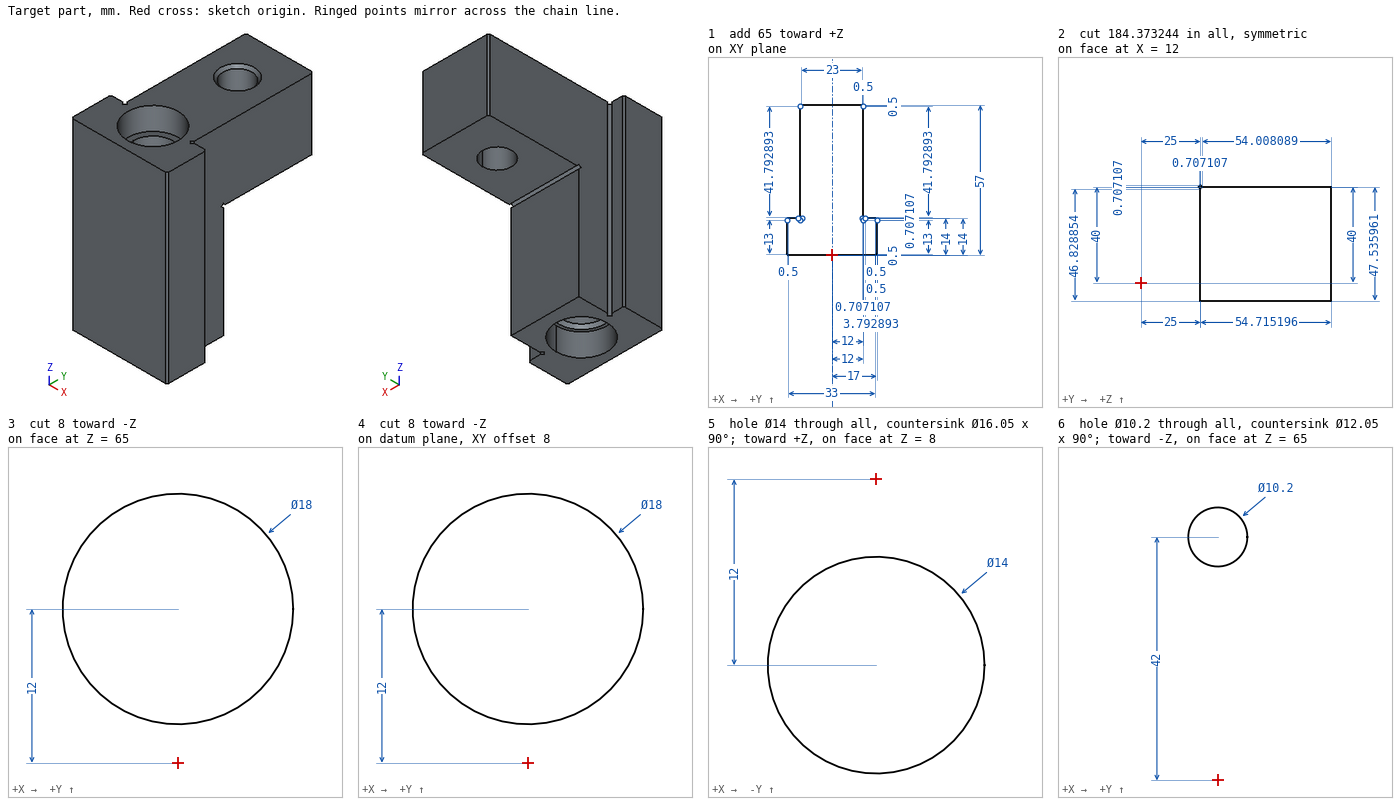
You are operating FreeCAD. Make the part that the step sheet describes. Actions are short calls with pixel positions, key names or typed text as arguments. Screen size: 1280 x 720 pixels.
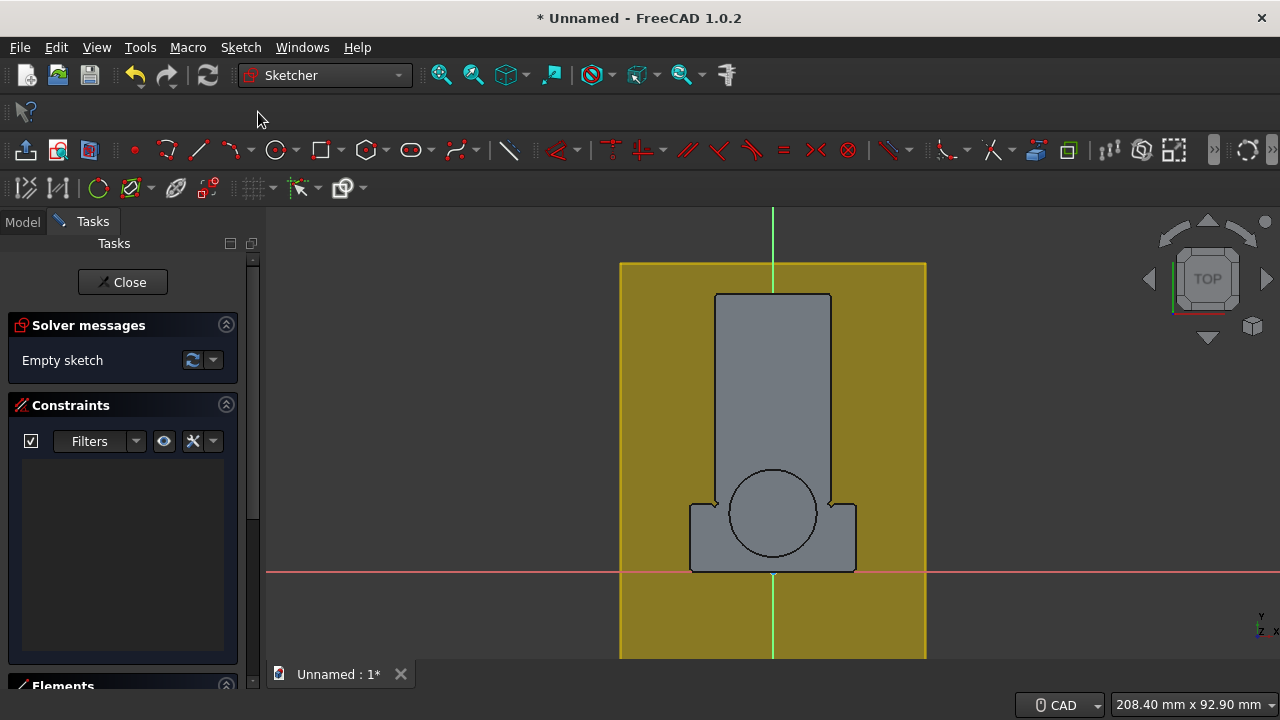
click(90, 150)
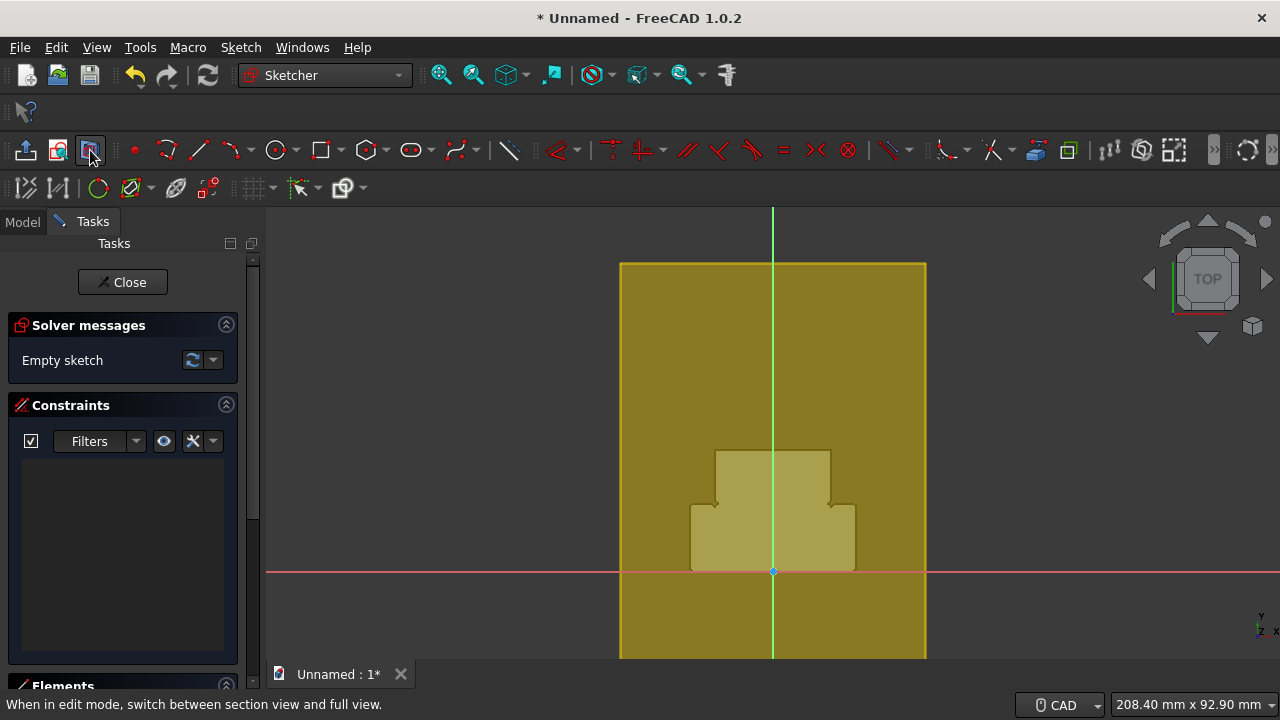
scroll(813, 572, up, 5)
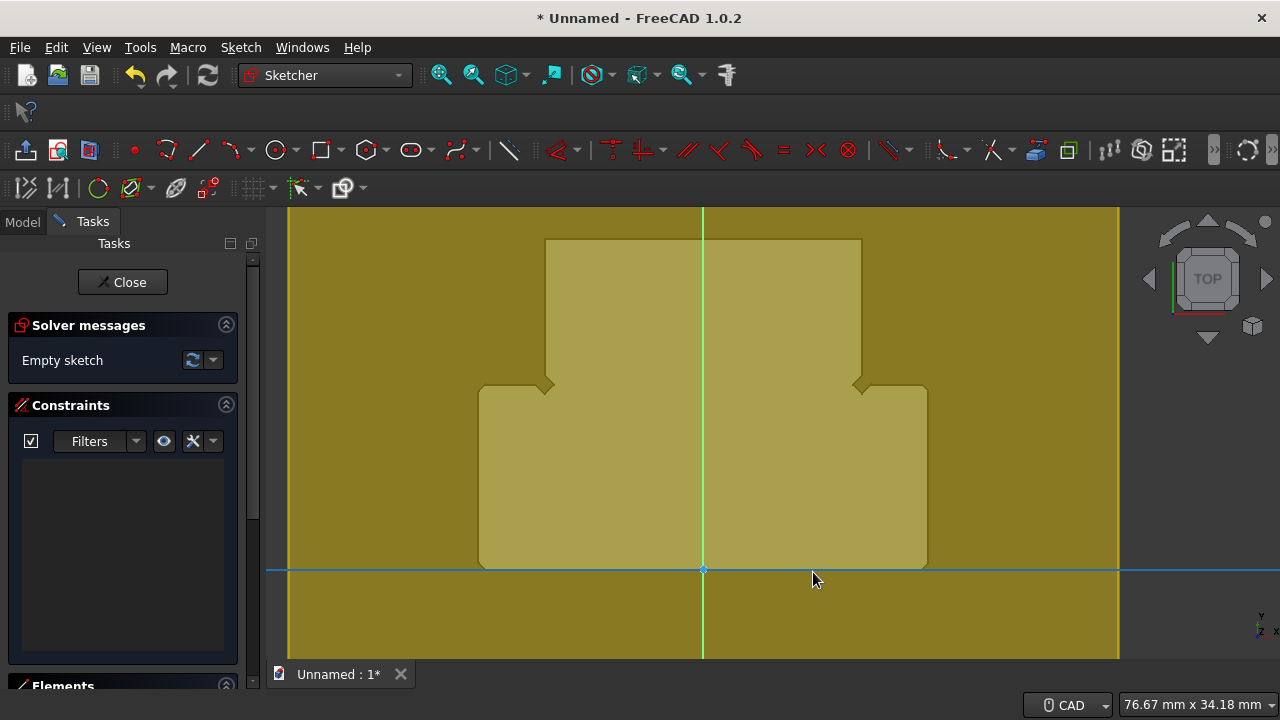
key(g)
key(c)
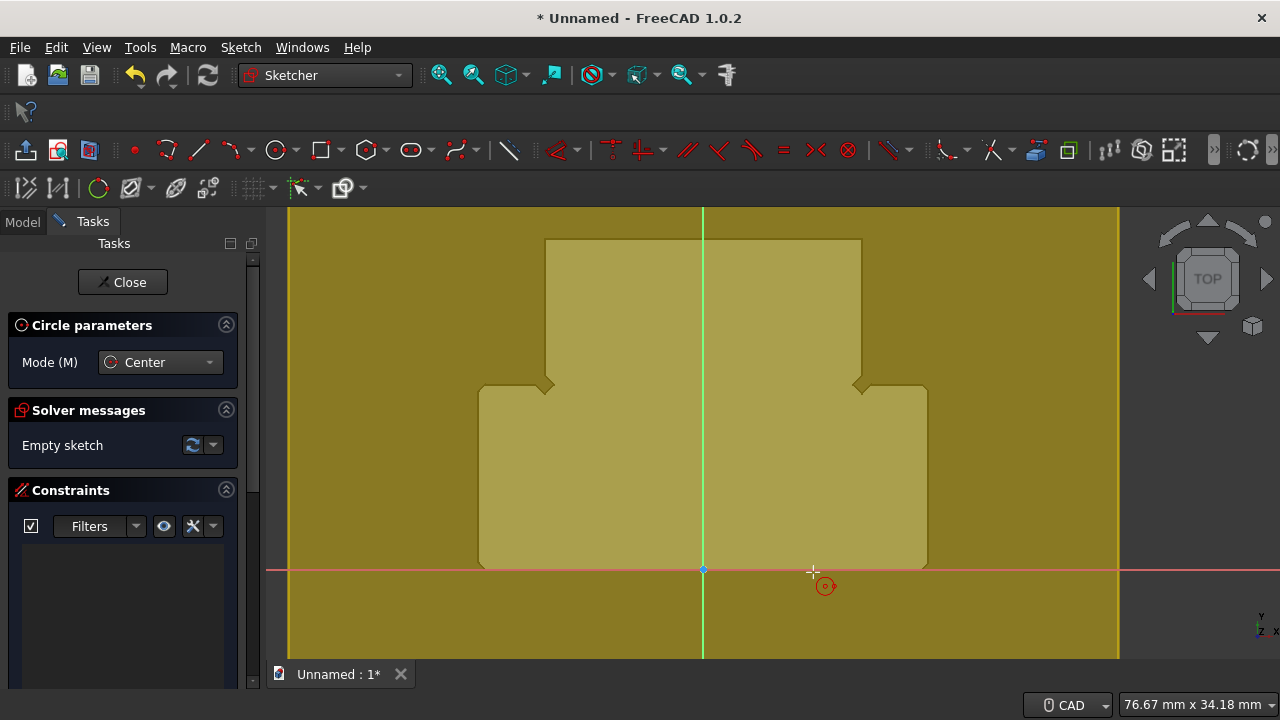
click(703, 411)
click(788, 327)
key(Escape)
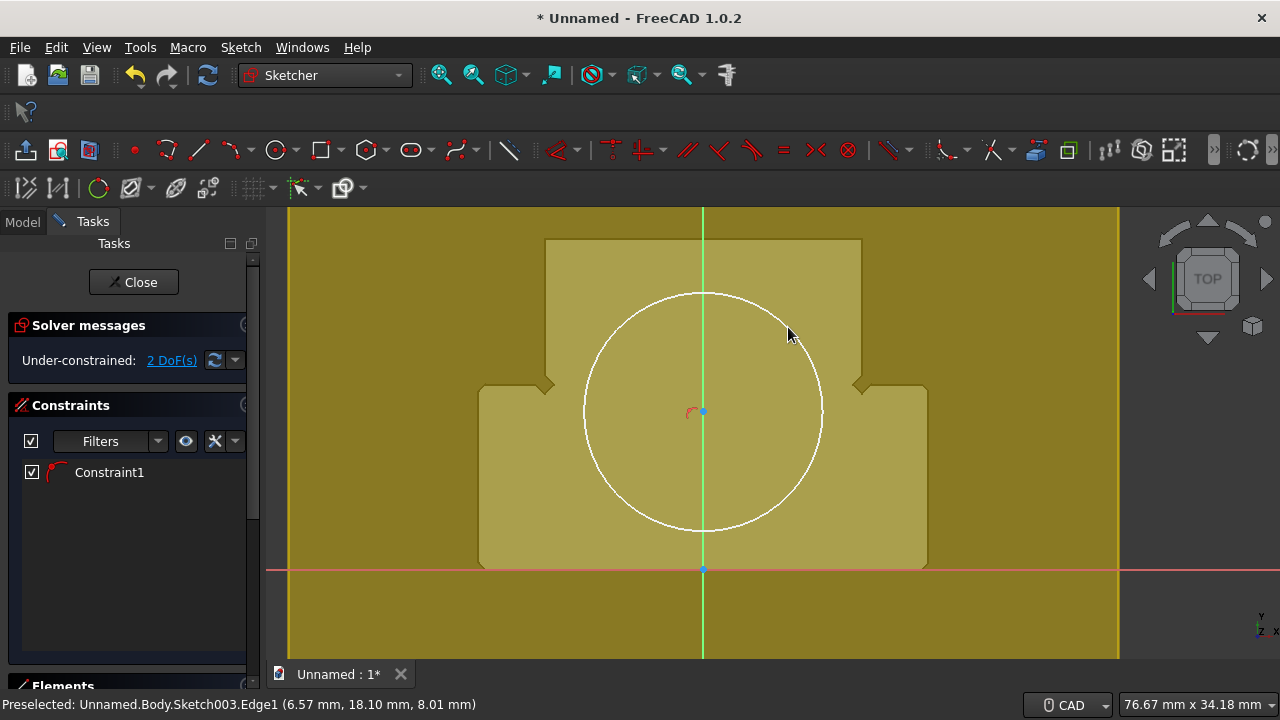
key(d)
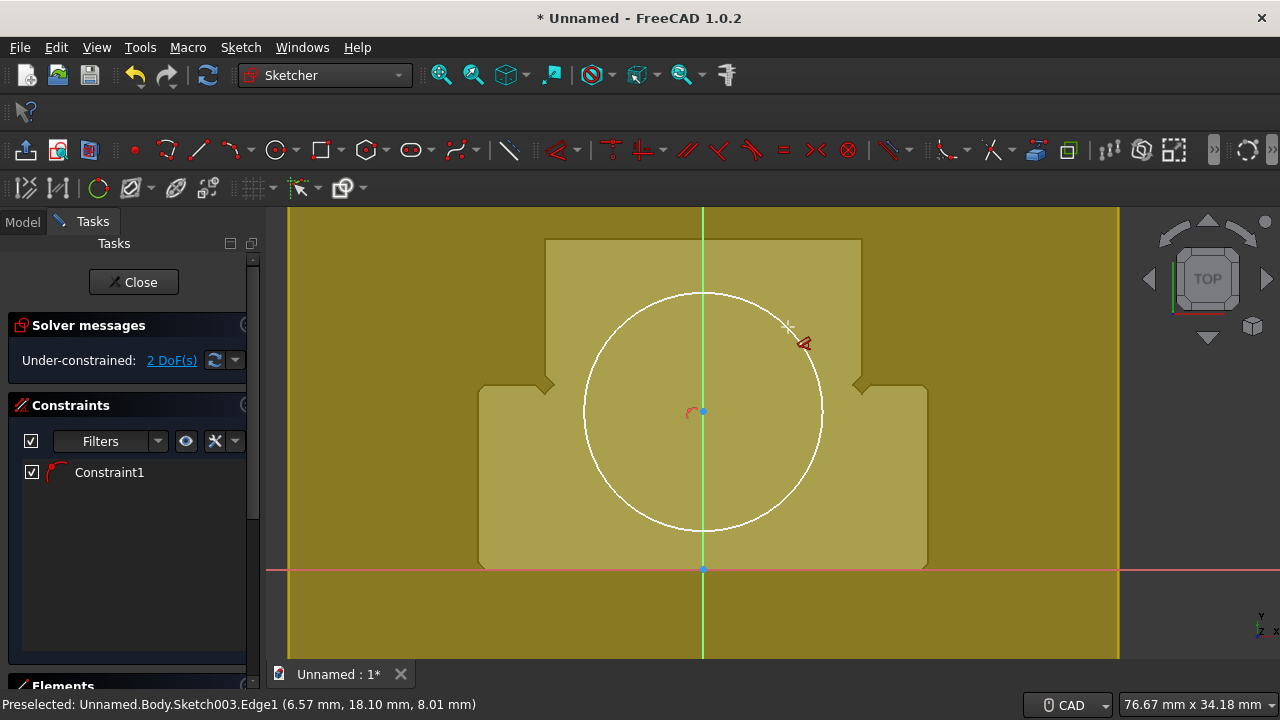
click(787, 327)
click(809, 304)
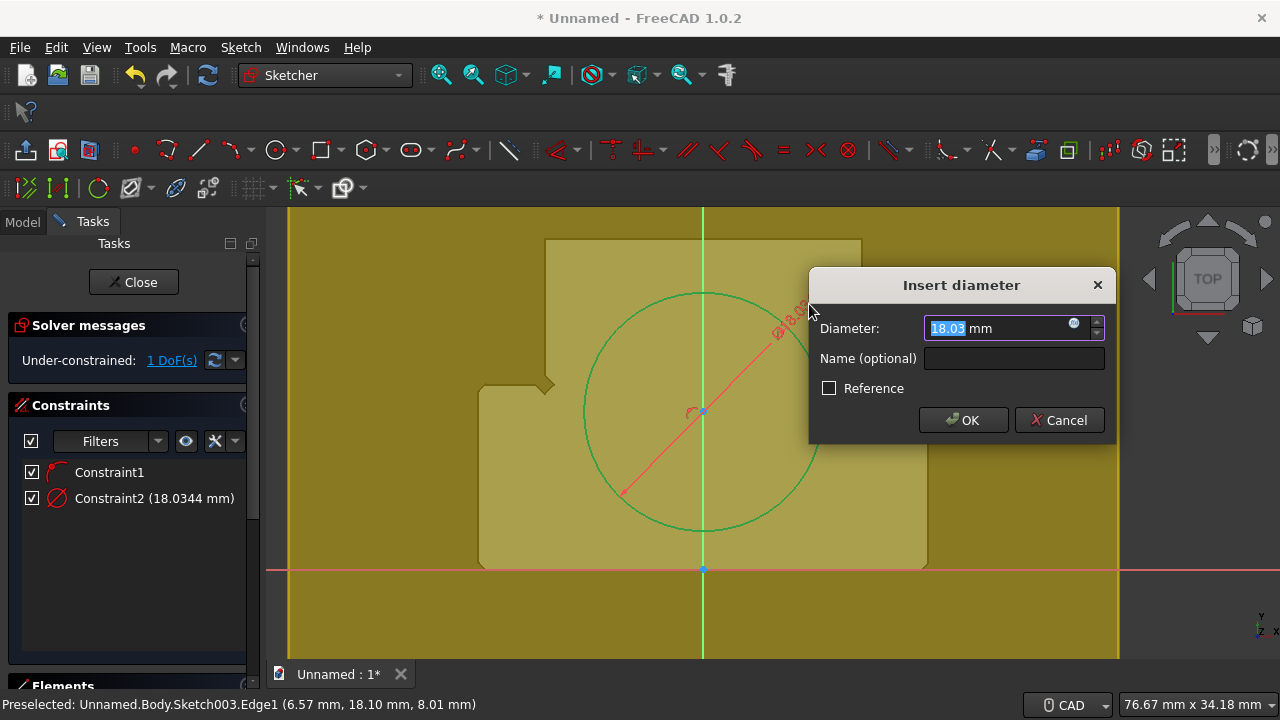
text(18)
key(Return)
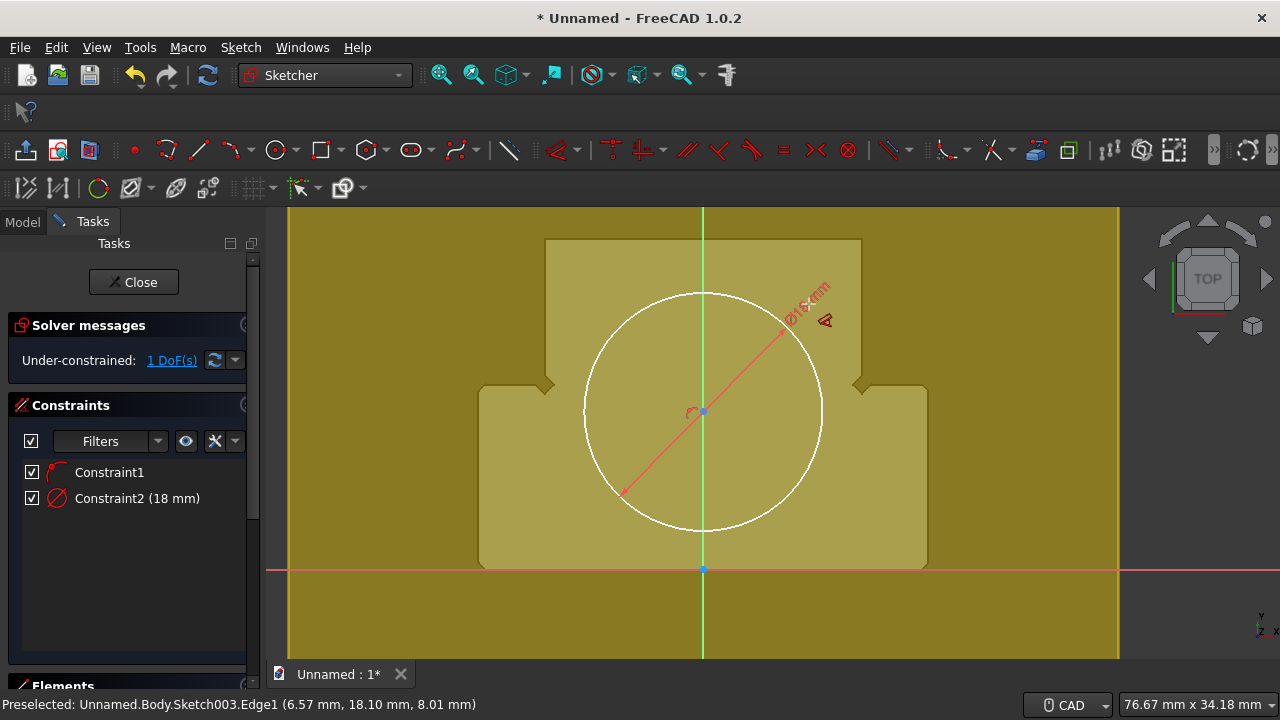
click(703, 412)
click(737, 491)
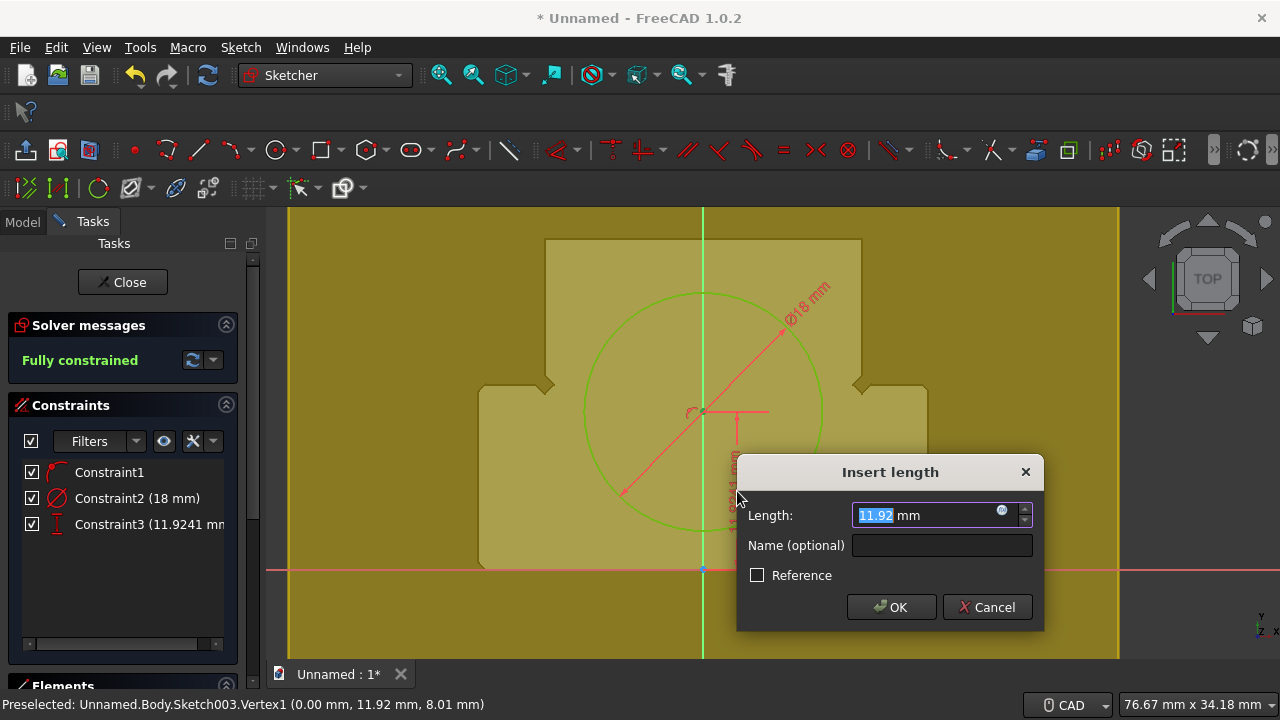
text(12)
key(Return)
key(Escape)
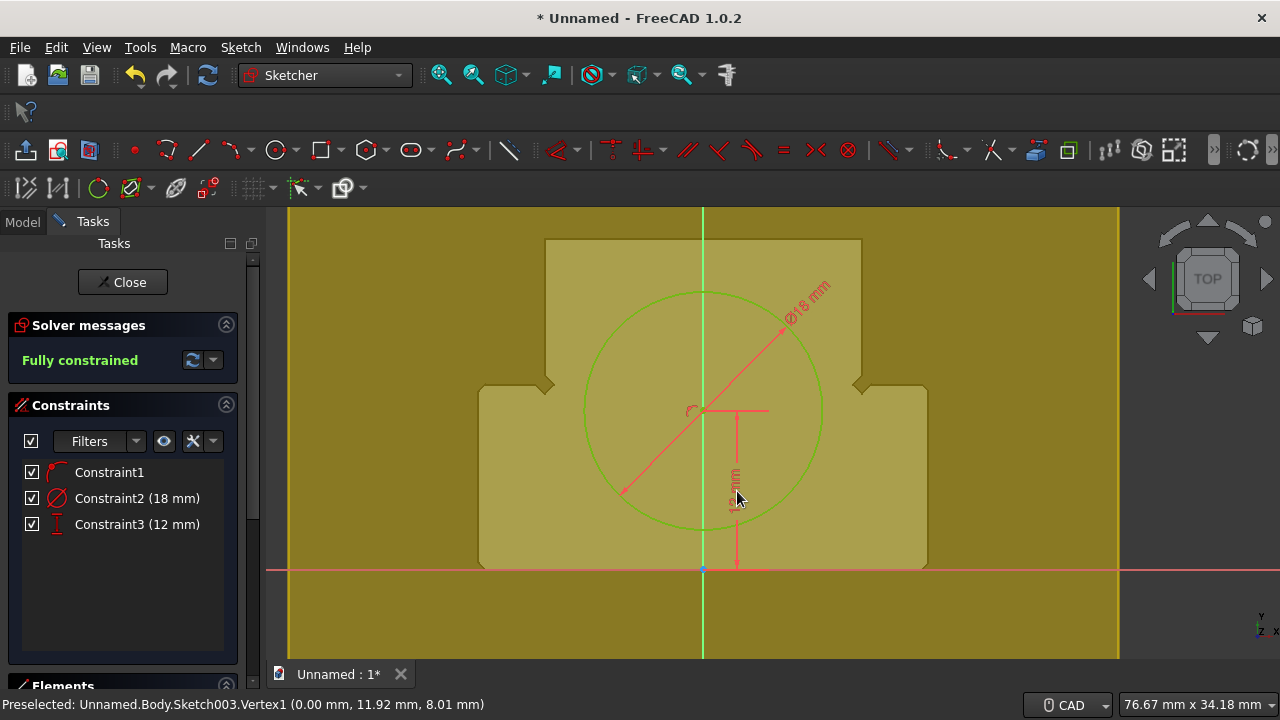
click(123, 282)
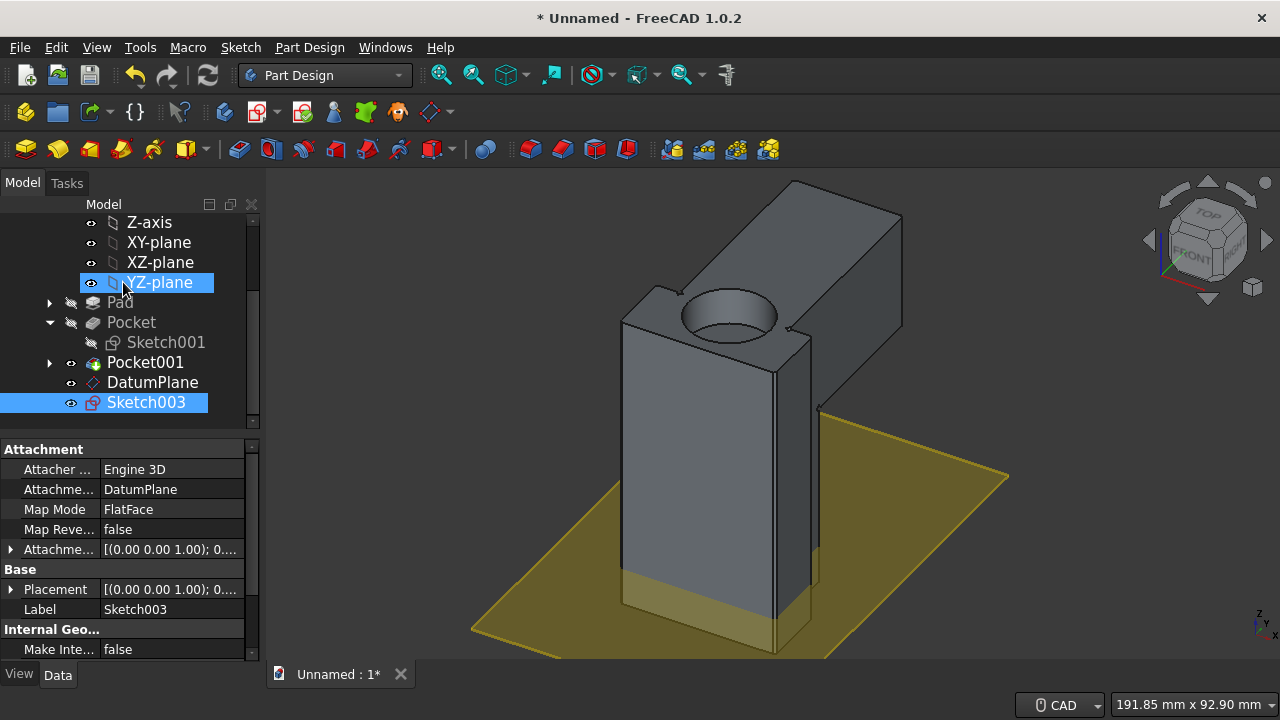
click(240, 150)